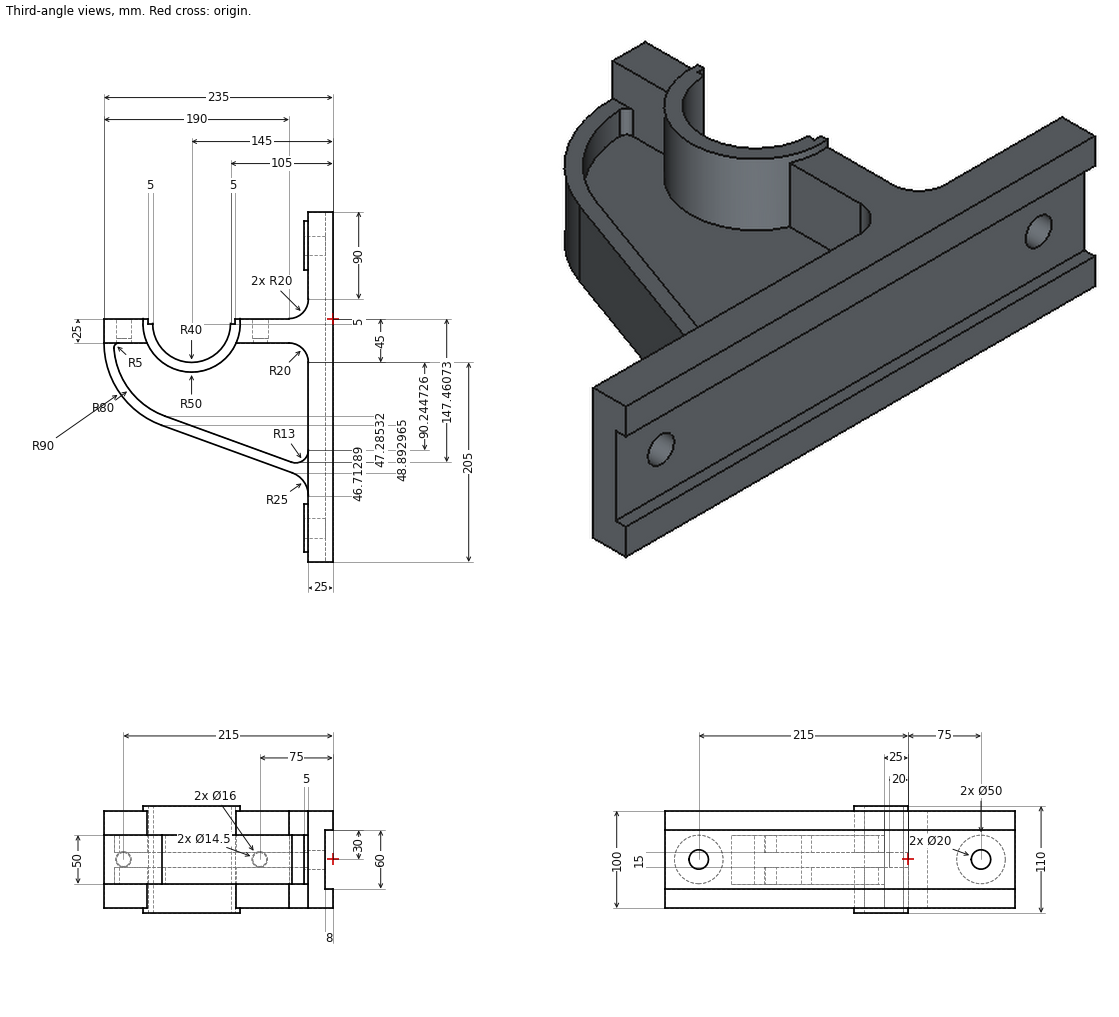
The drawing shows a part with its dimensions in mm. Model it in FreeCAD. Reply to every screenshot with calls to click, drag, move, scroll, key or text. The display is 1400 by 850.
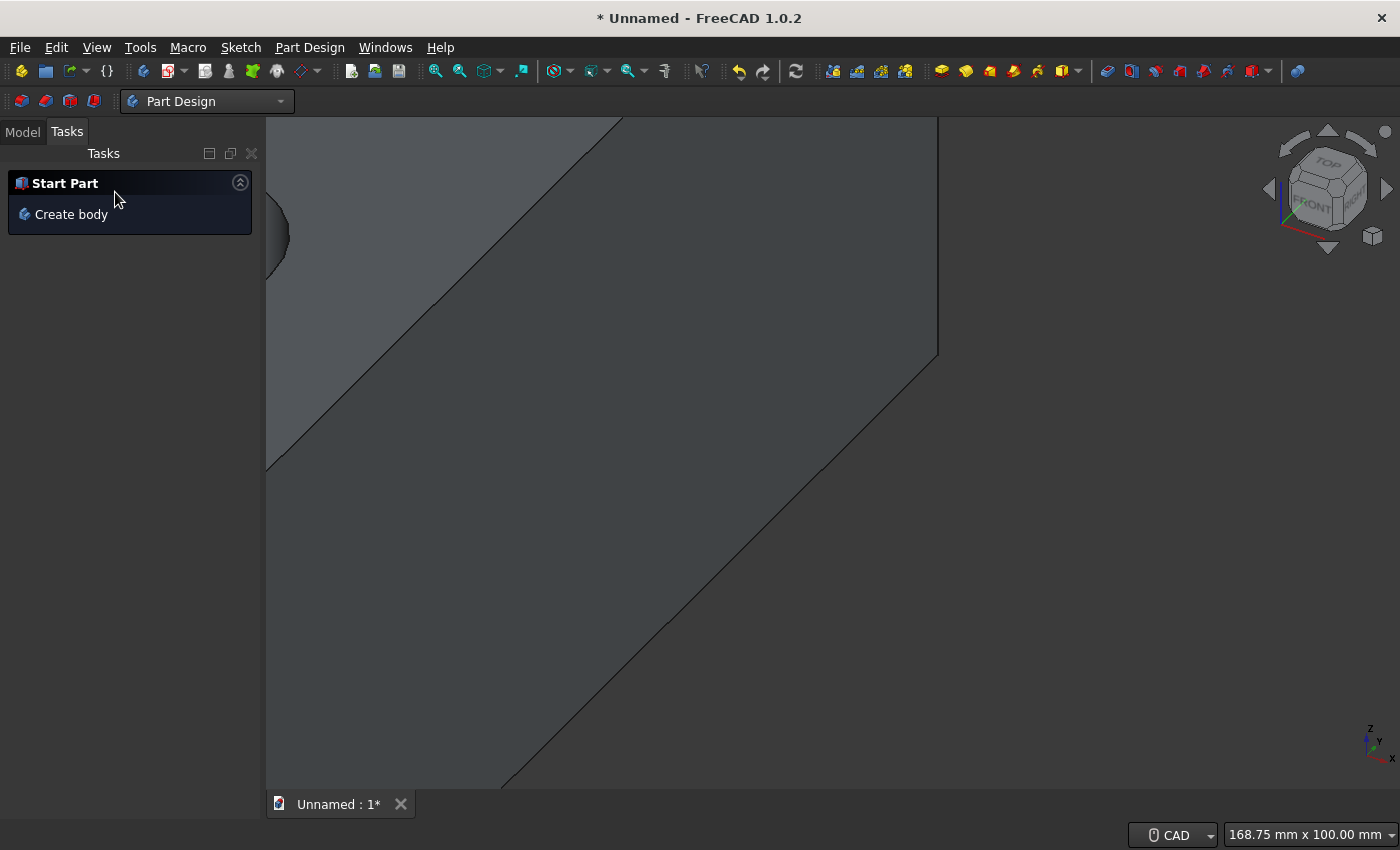
click(436, 72)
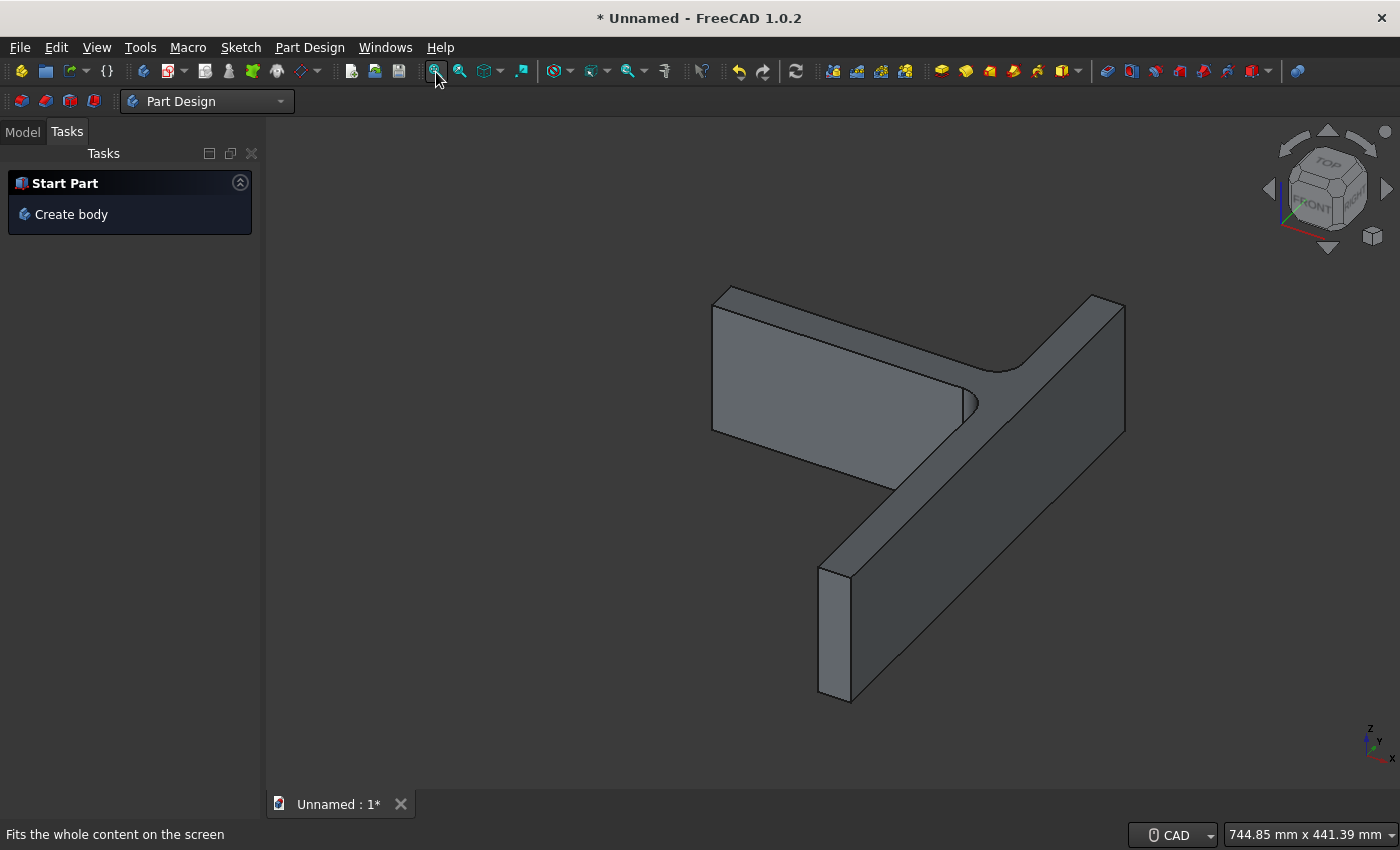
key(4)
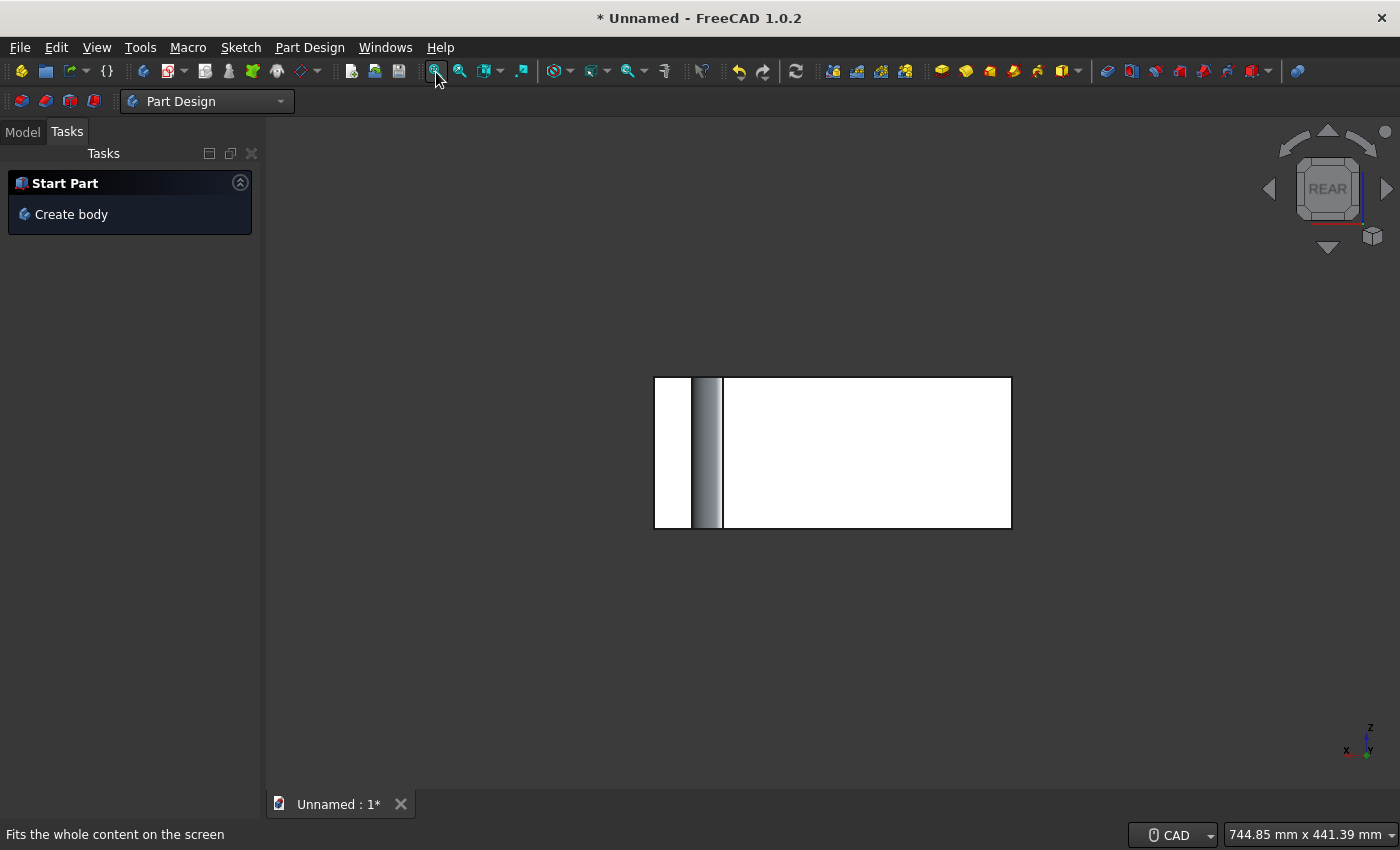
click(436, 72)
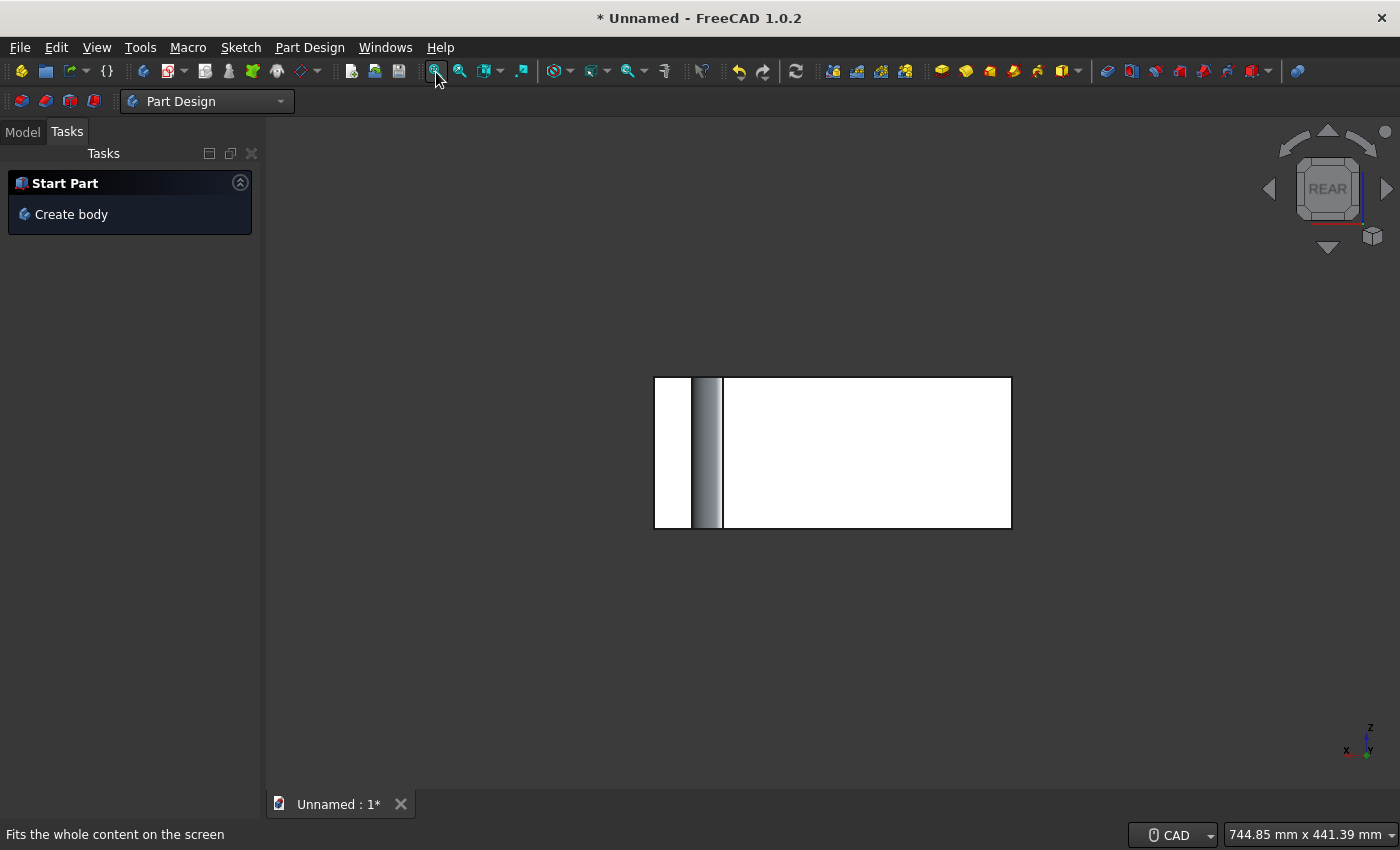
click(673, 409)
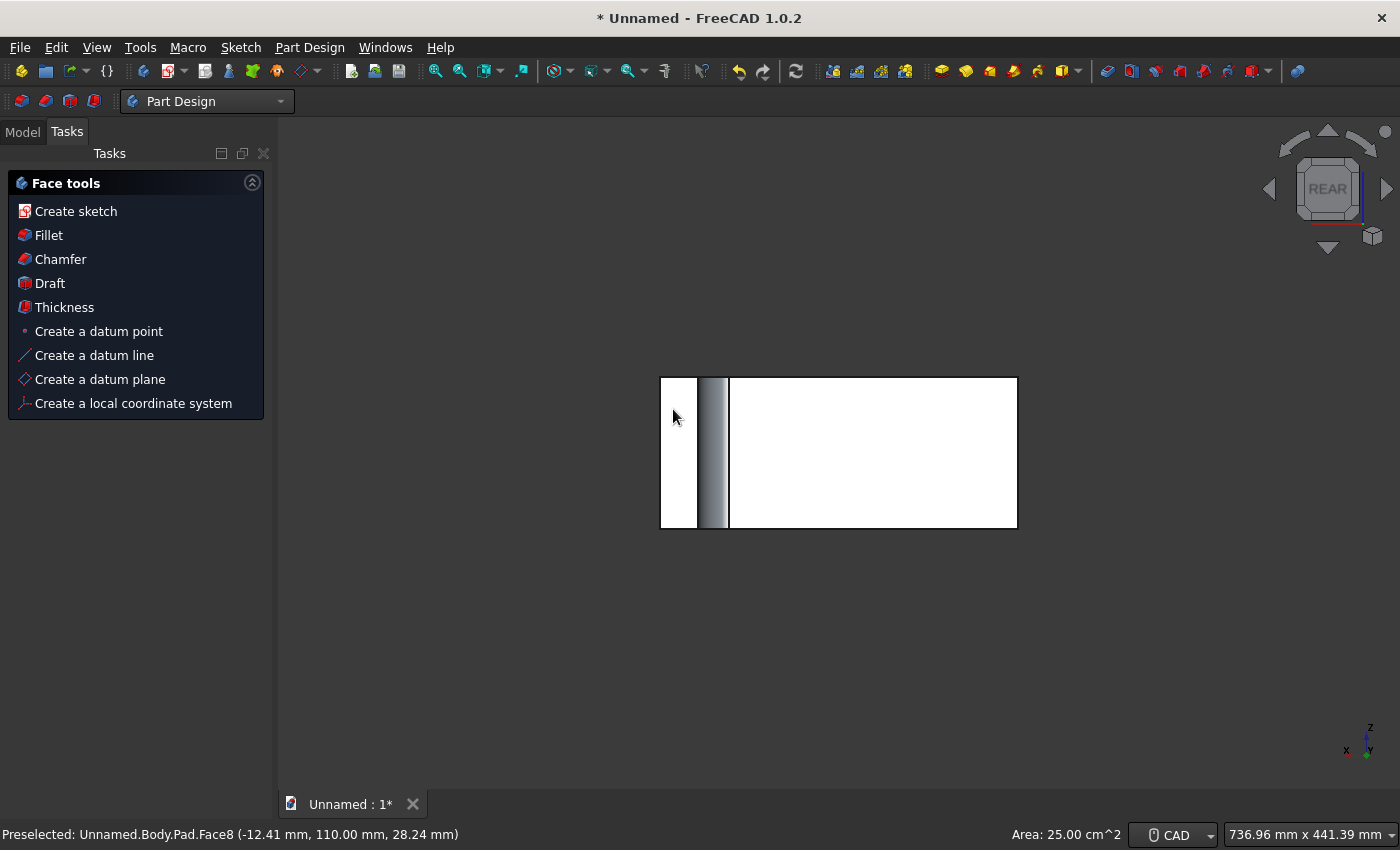
click(168, 72)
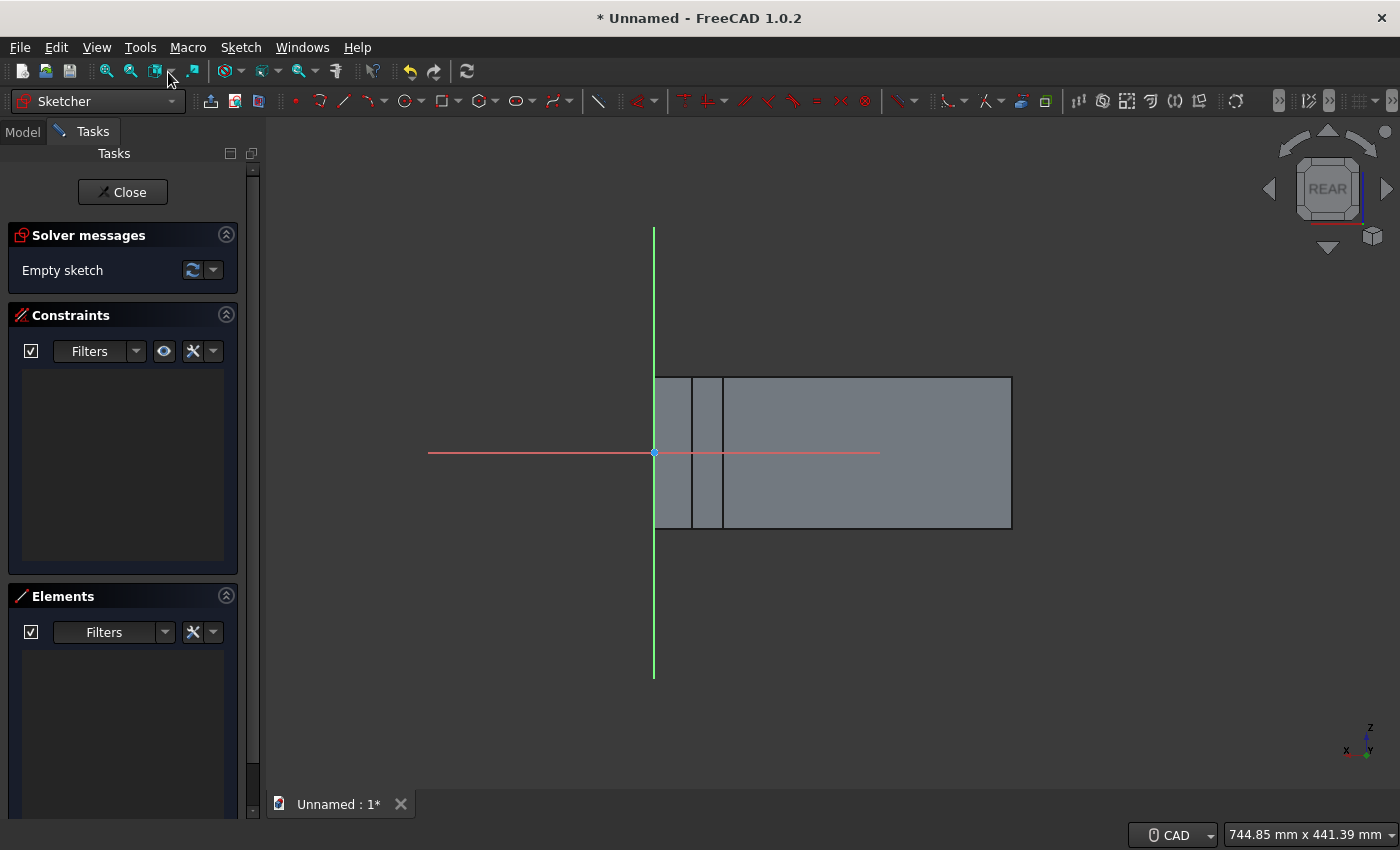
scroll(634, 453, up, 8)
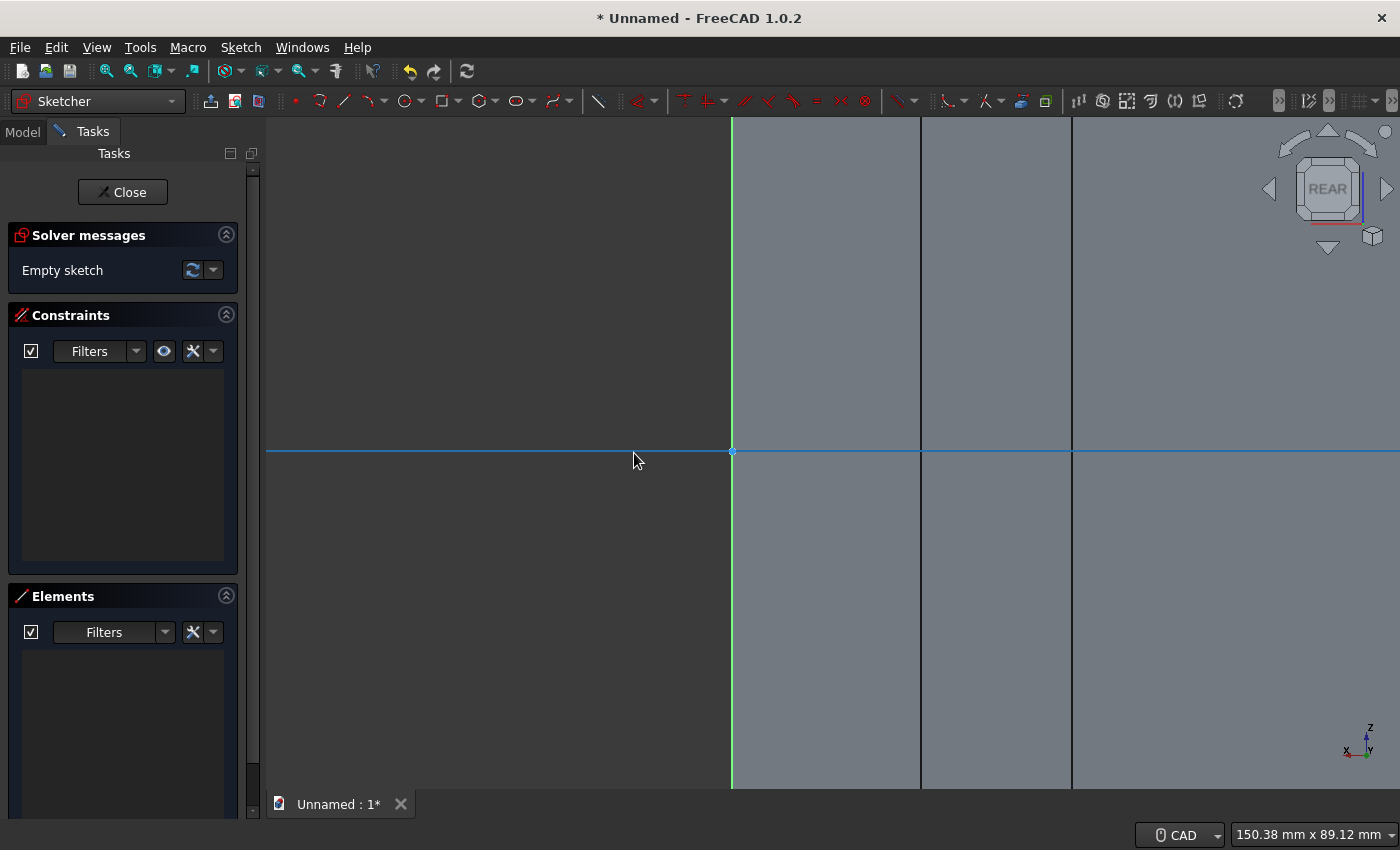
click(442, 102)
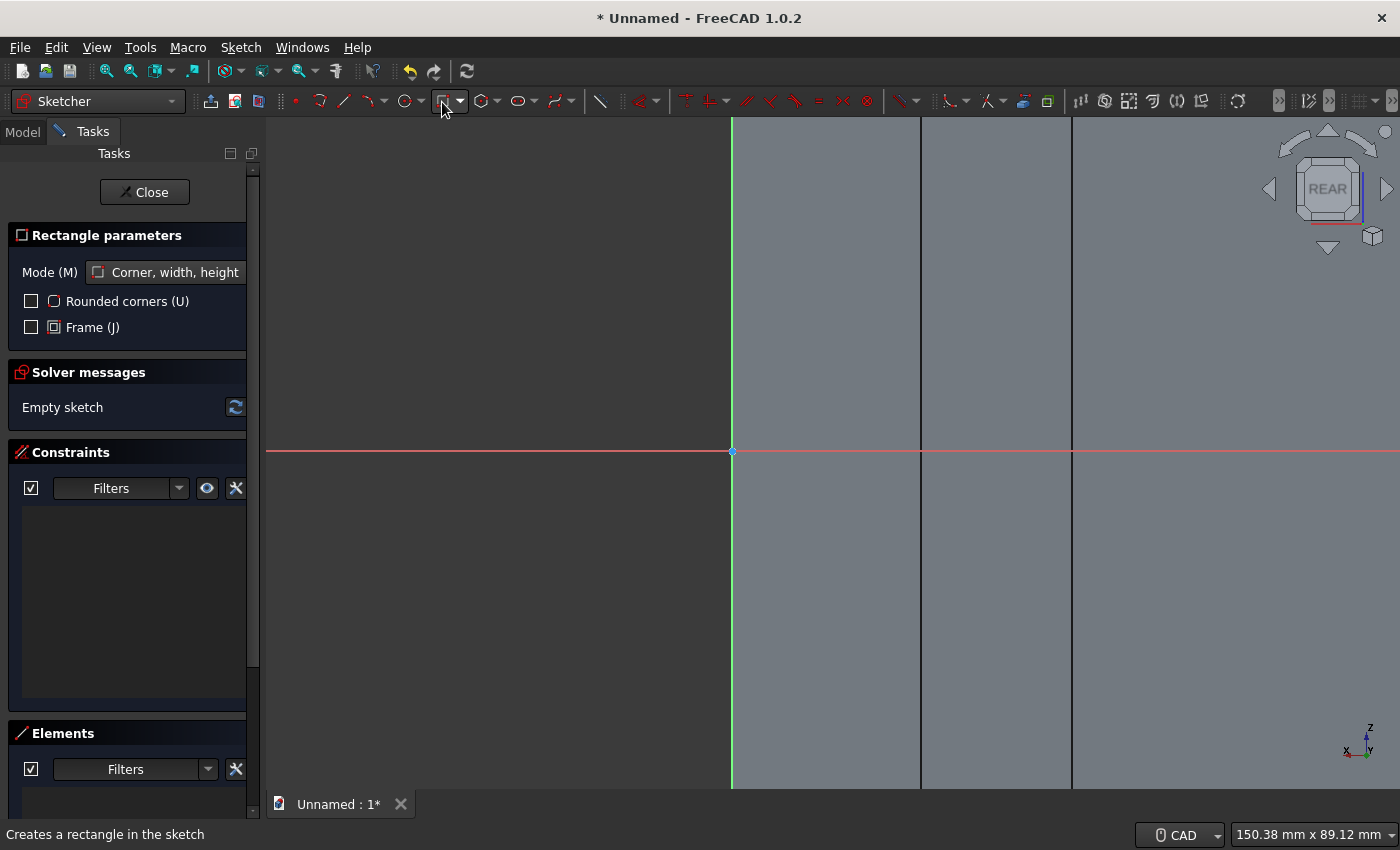
click(732, 225)
move(793, 677)